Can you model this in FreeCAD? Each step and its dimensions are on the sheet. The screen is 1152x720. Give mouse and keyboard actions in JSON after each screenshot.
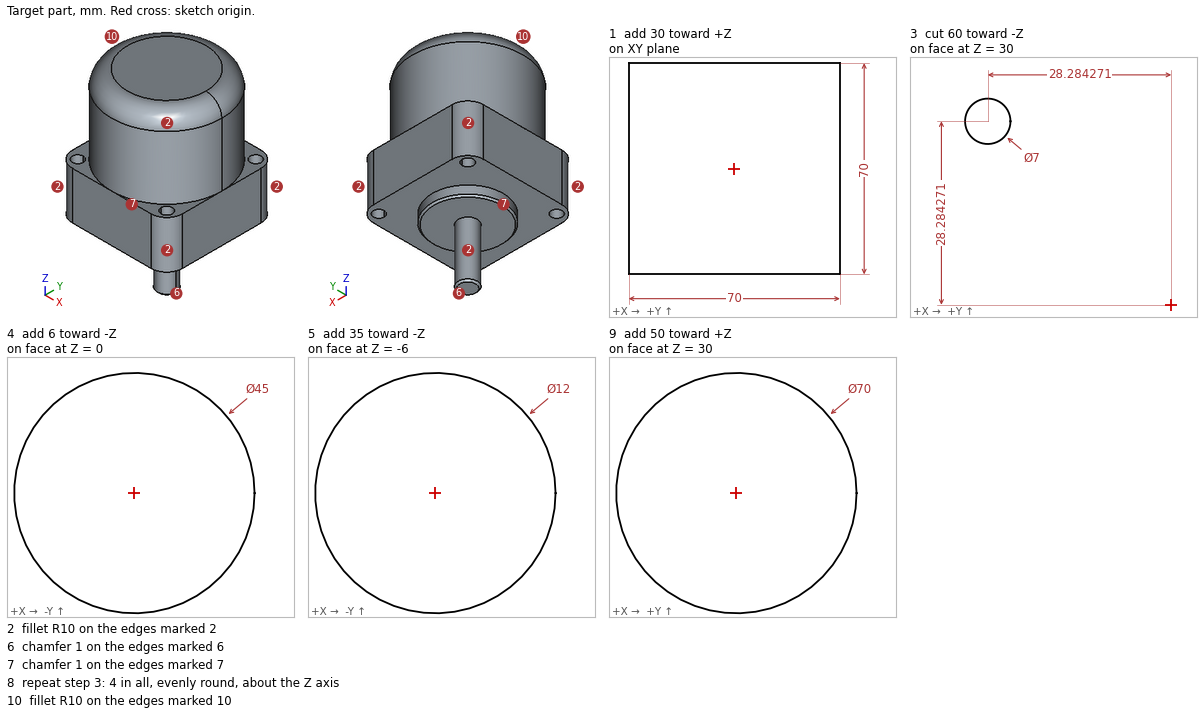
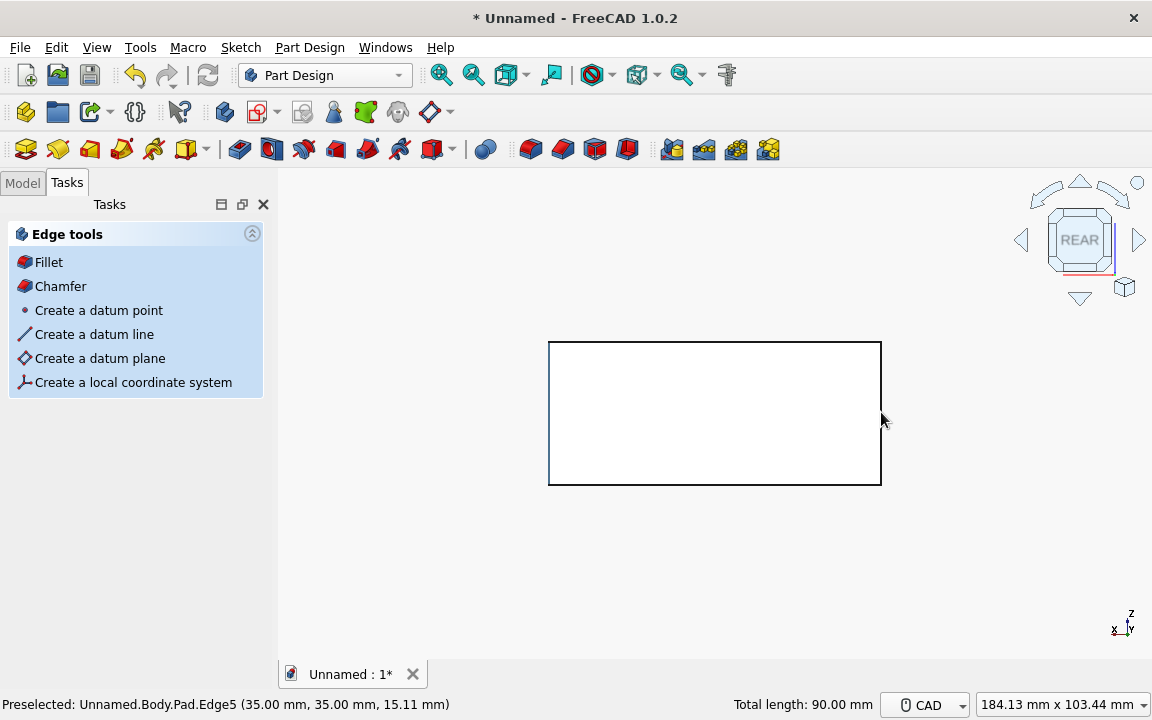
{"action": "left_click", "coordinate": [881, 413], "text": "ctrl"}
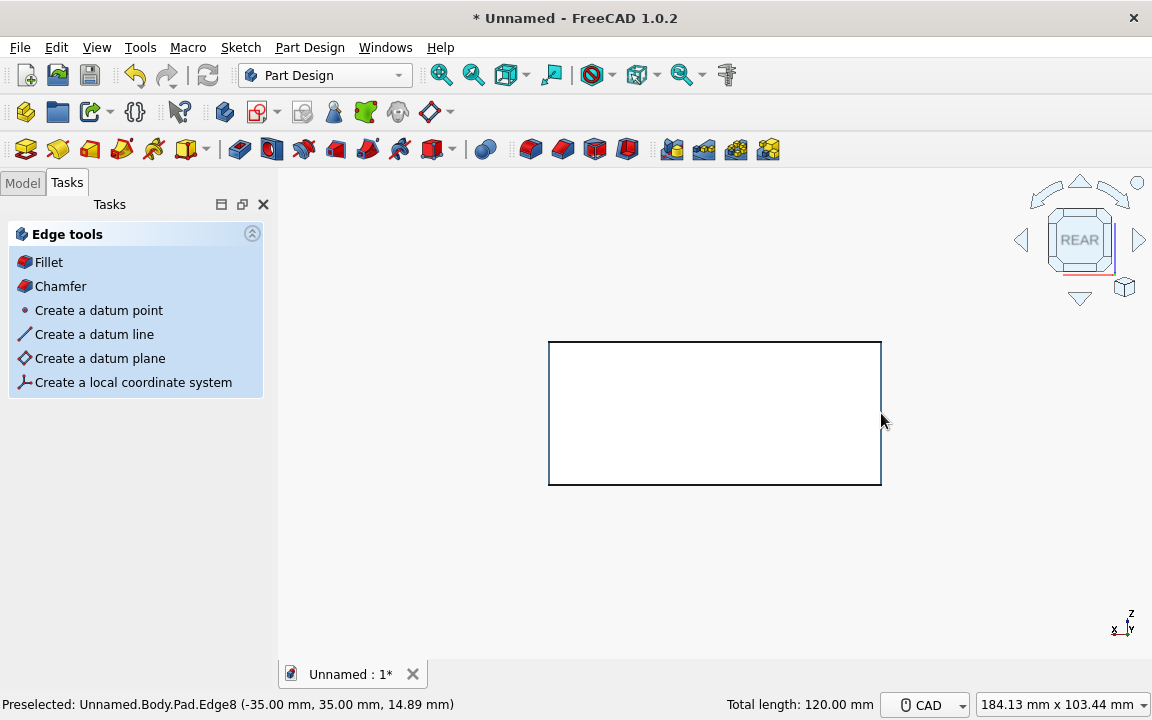
{"action": "left_click", "coordinate": [532, 150]}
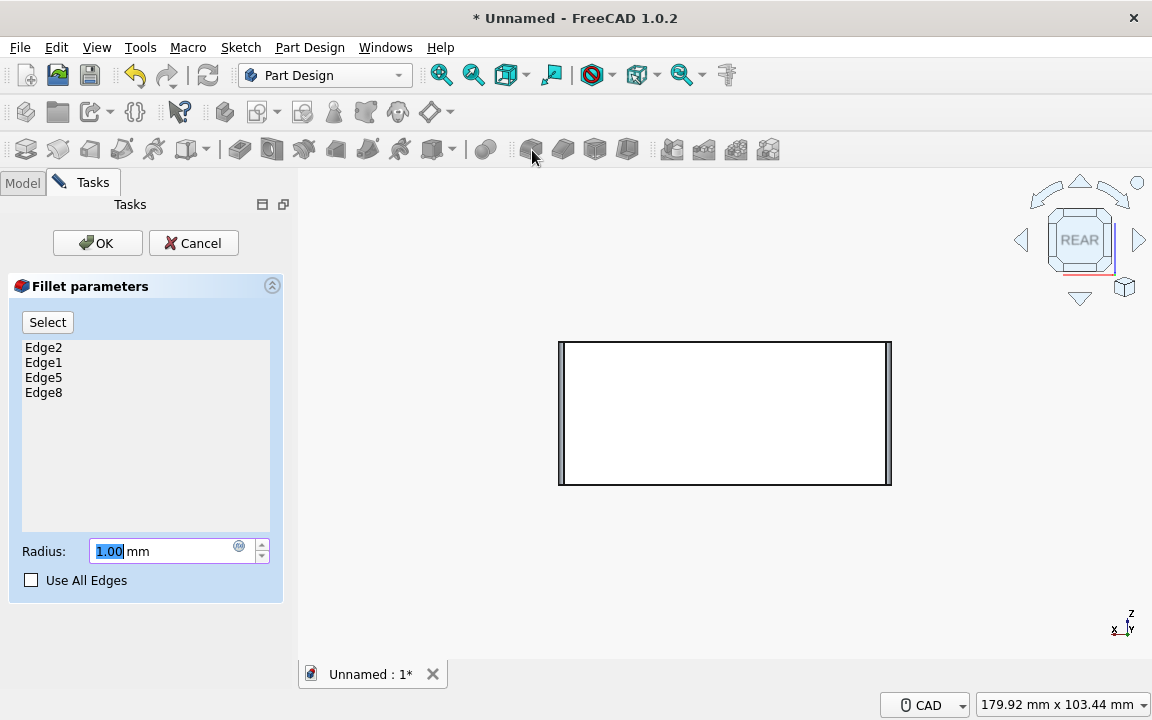
{"action": "type", "text": "10"}
{"action": "key", "text": "Tab"}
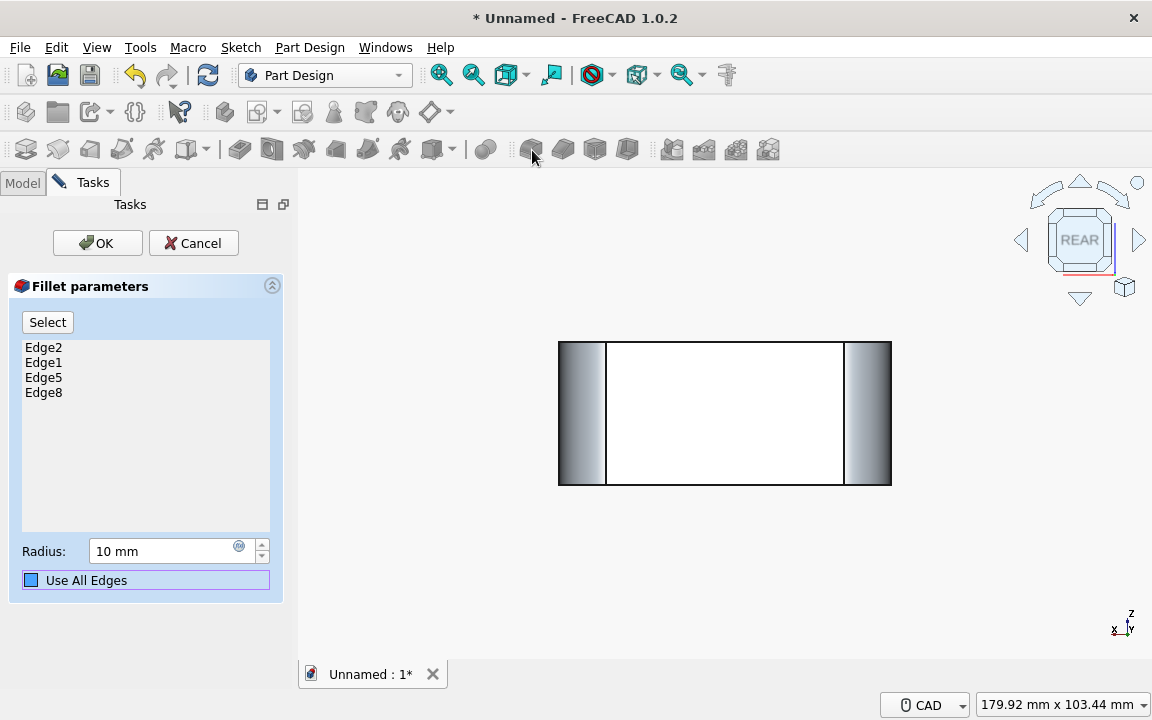
{"action": "left_click", "coordinate": [98, 243]}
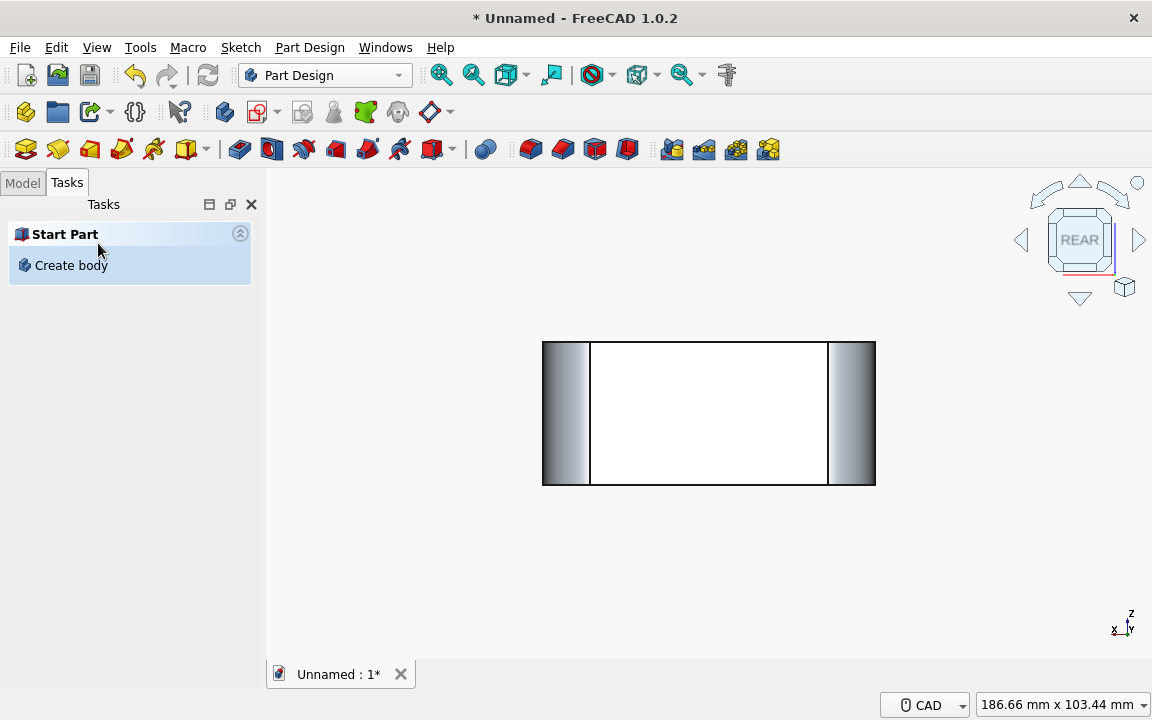
{"action": "left_click", "coordinate": [442, 76]}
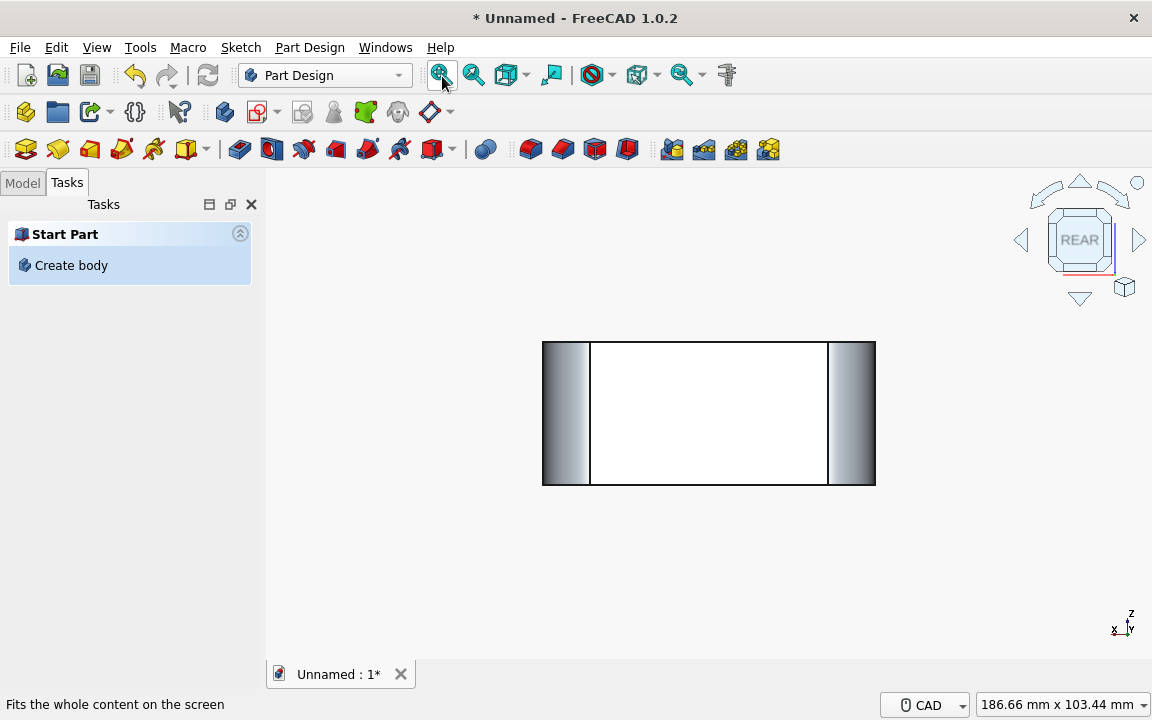
{"action": "key", "text": "0"}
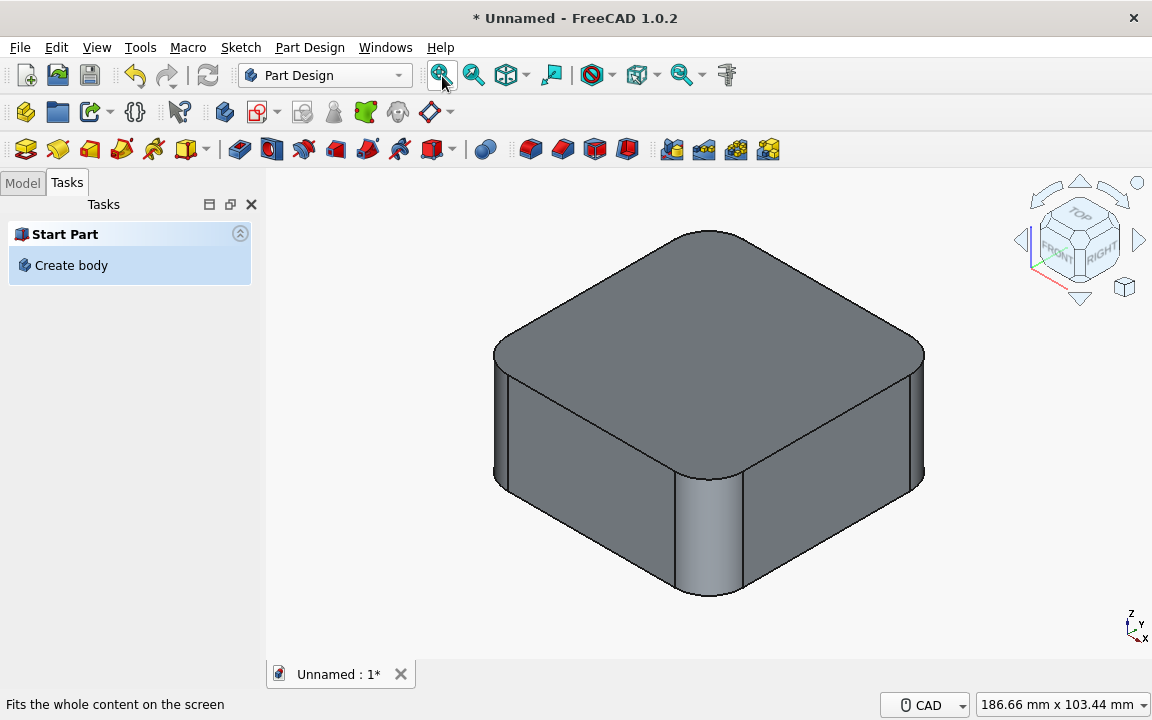
{"action": "left_click", "coordinate": [709, 354]}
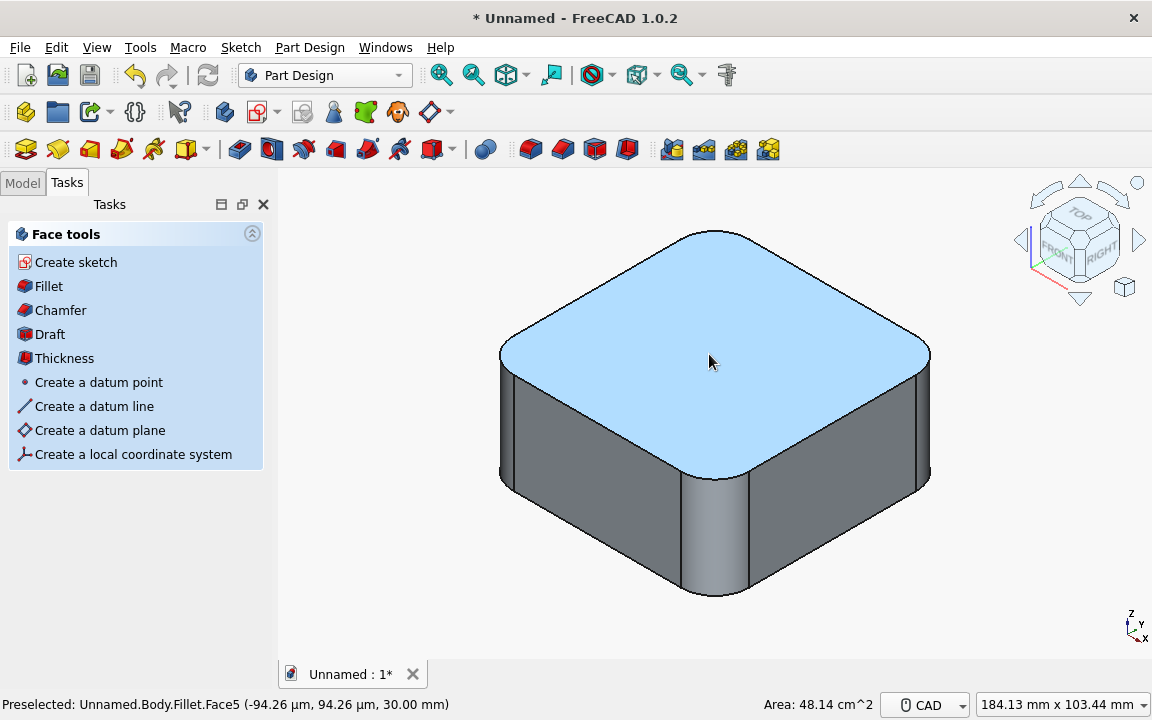
{"action": "left_click", "coordinate": [258, 112]}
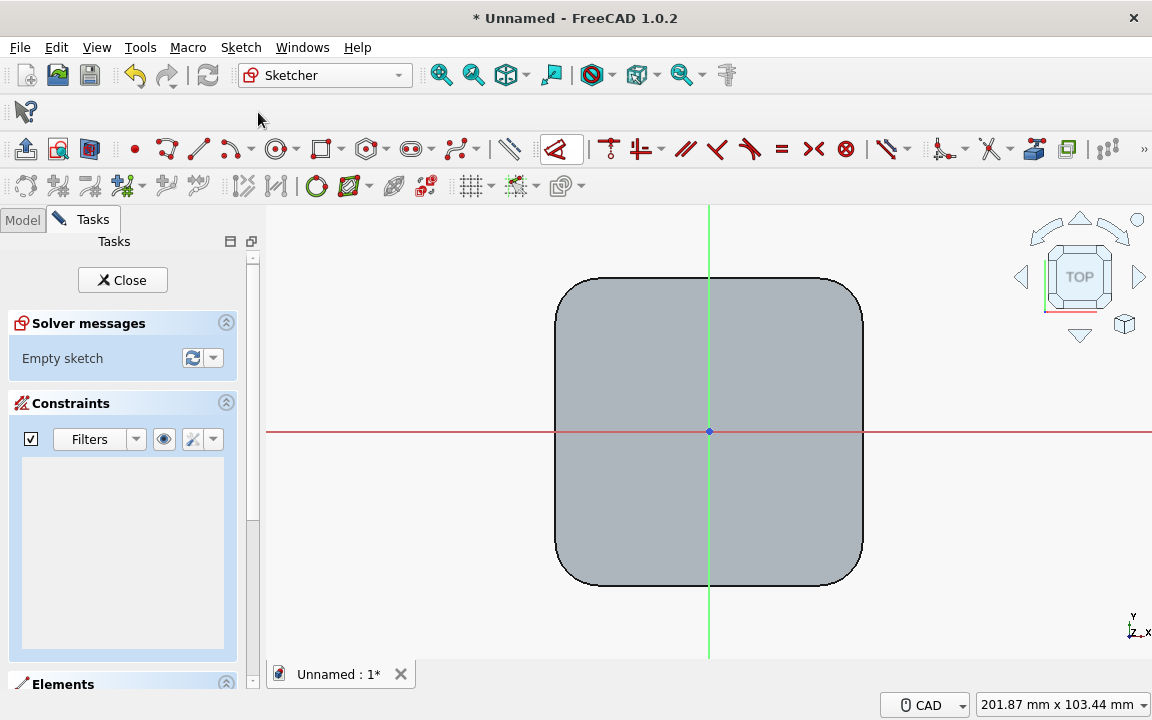
{"action": "scroll", "coordinate": [578, 292], "scroll_direction": "up", "scroll_amount": 11}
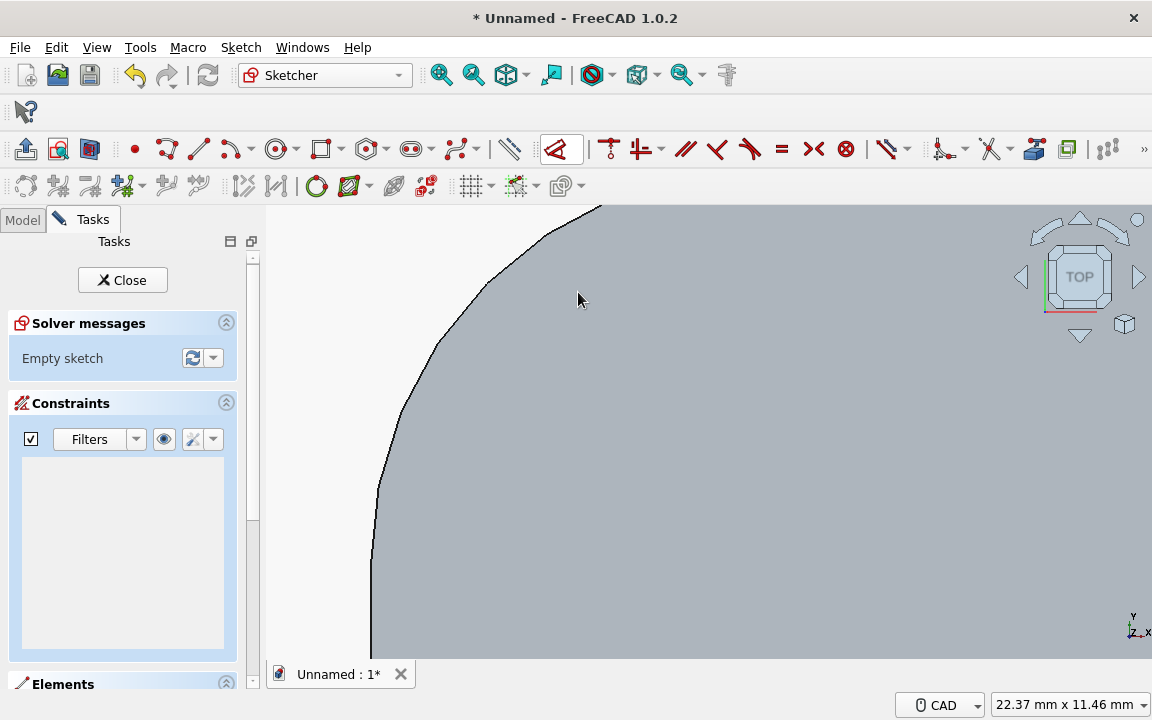
{"action": "key", "text": "g c"}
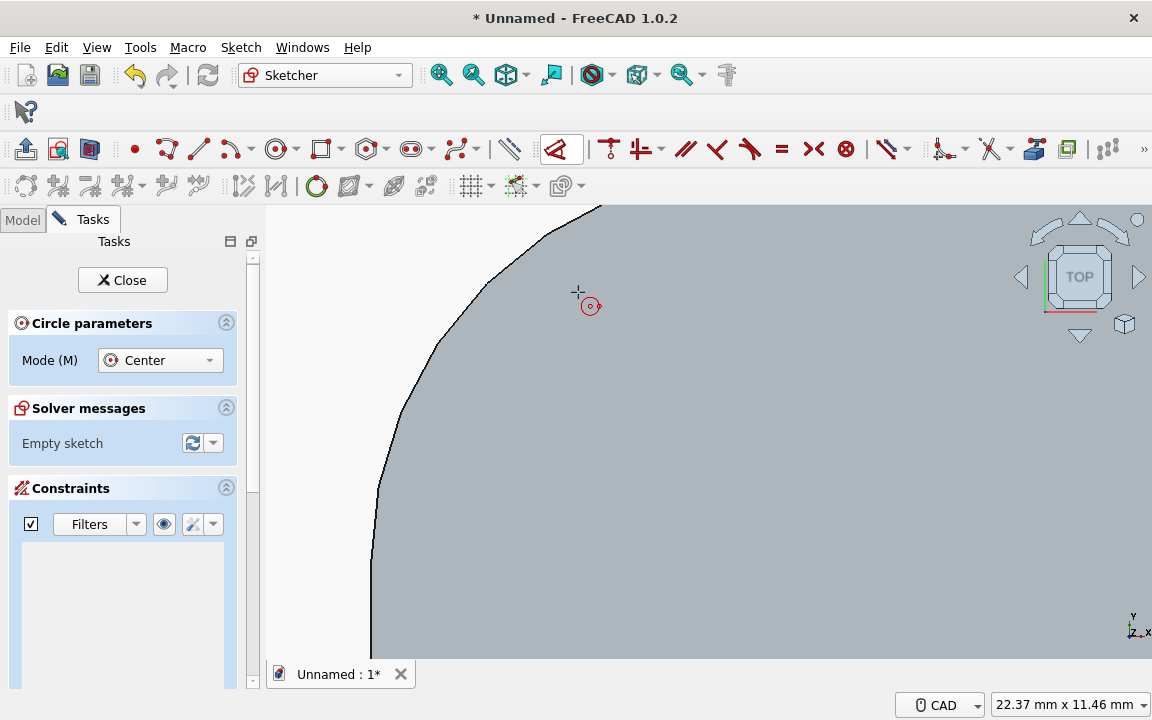
{"action": "left_click", "coordinate": [637, 434]}
{"action": "mouse_move", "coordinate": [735, 336]}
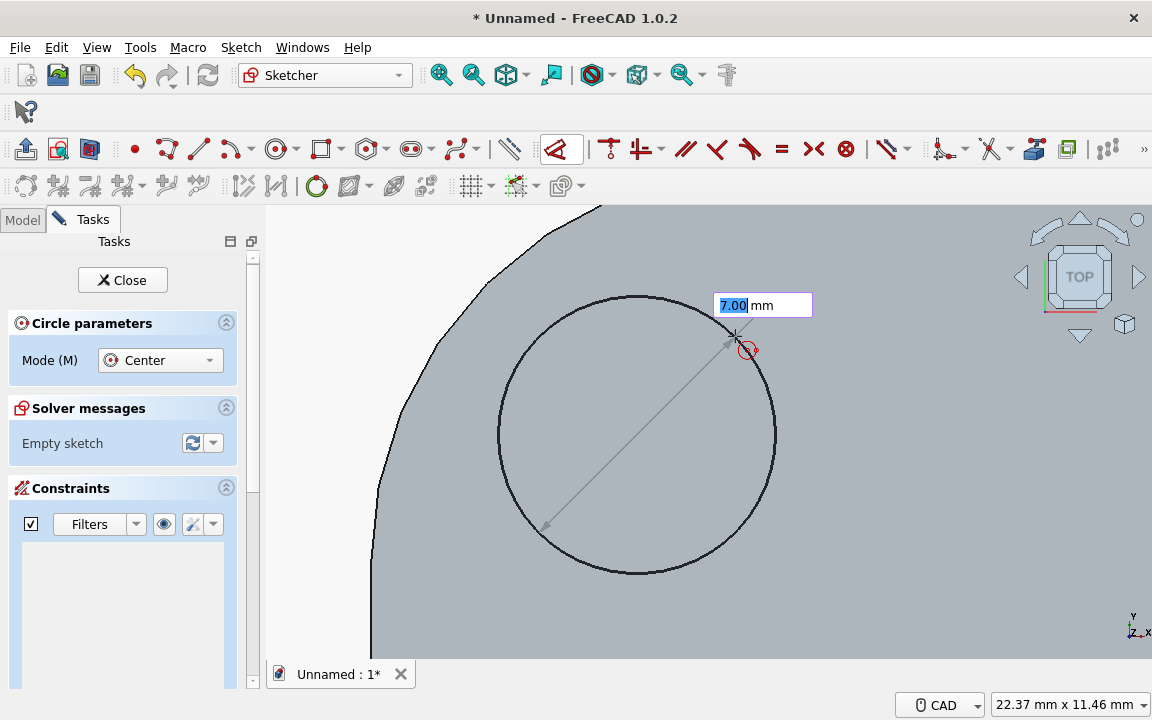
{"action": "type", "text": "7"}
{"action": "key", "text": "Return"}
{"action": "key", "text": "Escape"}